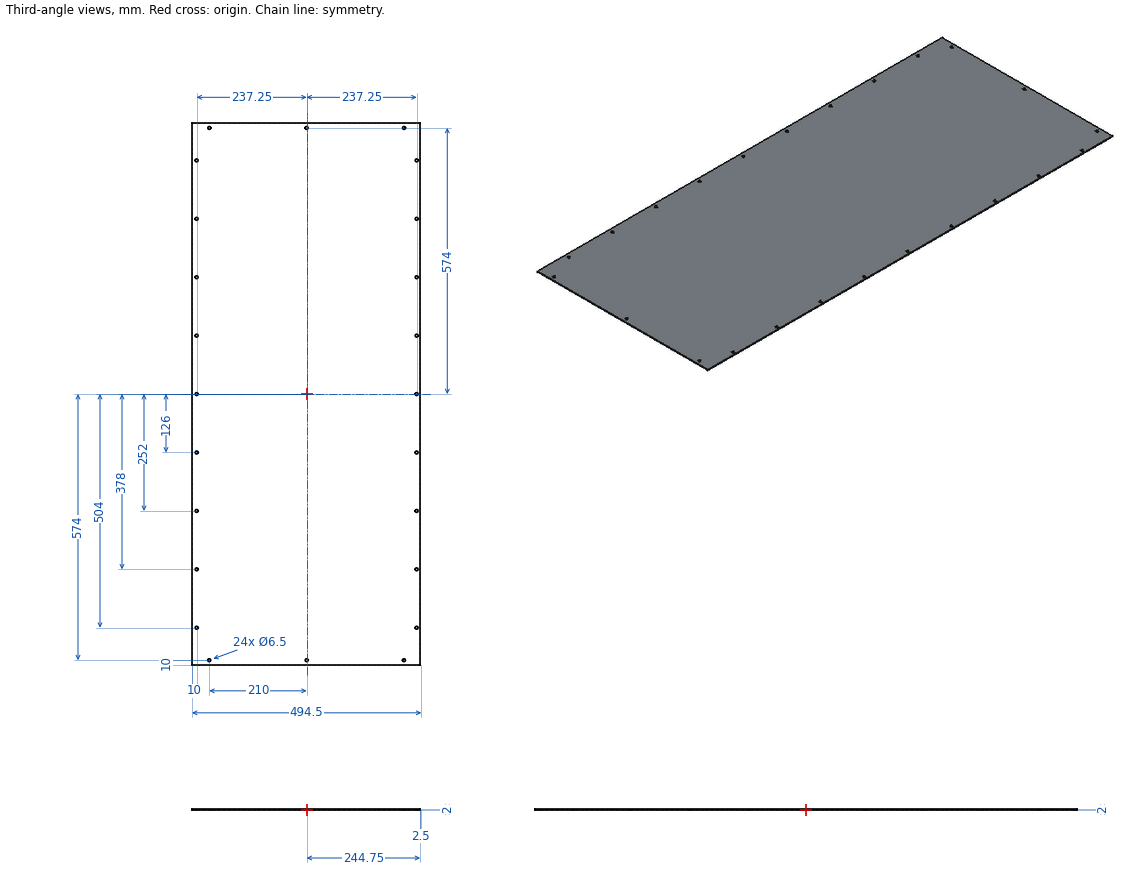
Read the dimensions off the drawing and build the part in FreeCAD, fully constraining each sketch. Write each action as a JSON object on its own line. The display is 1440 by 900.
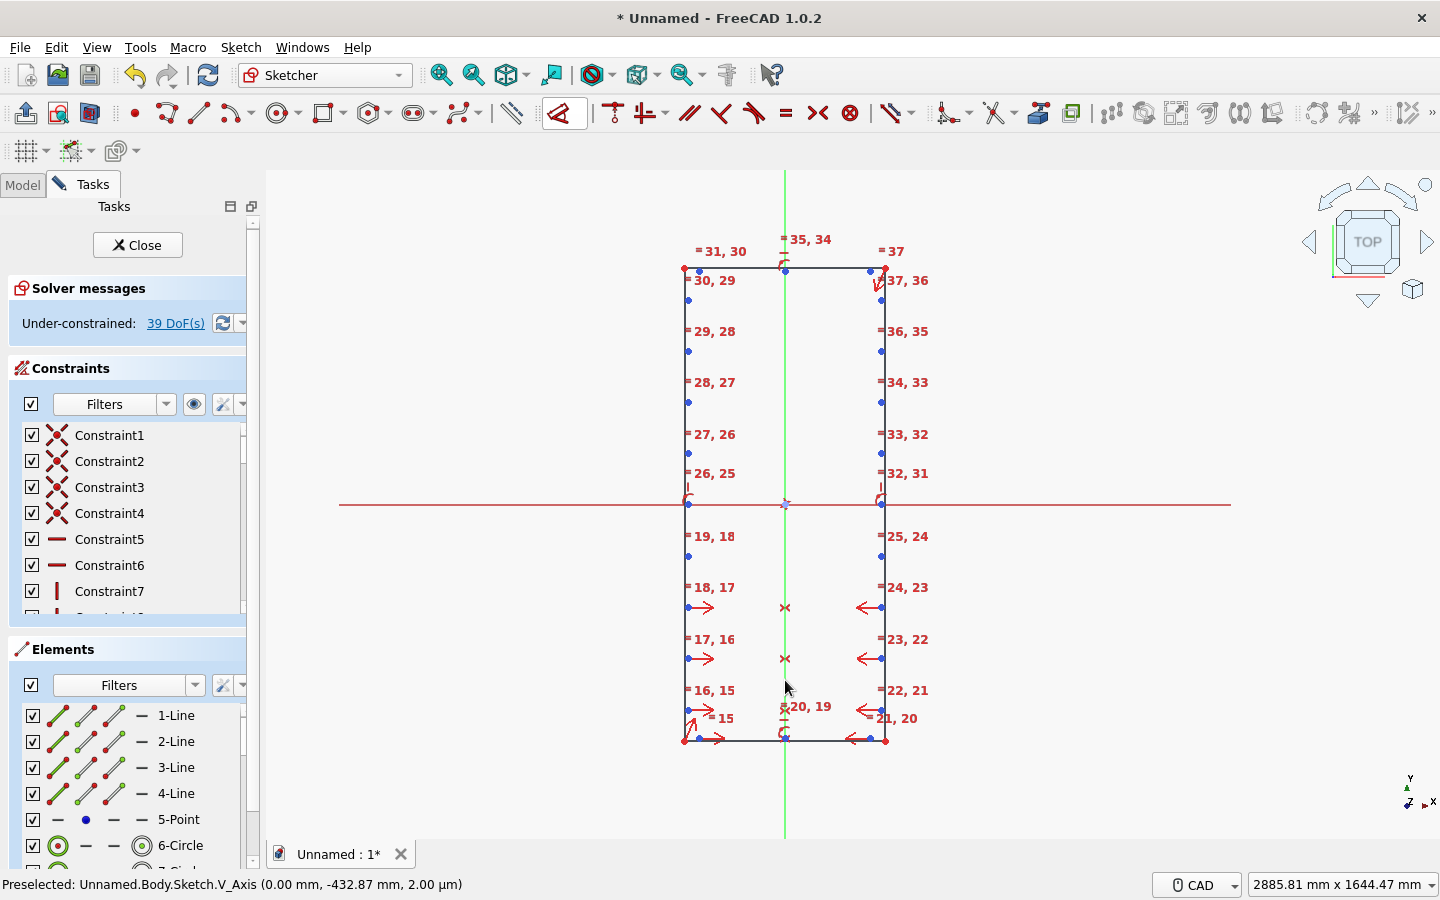
{"action": "left_click", "coordinate": [689, 556]}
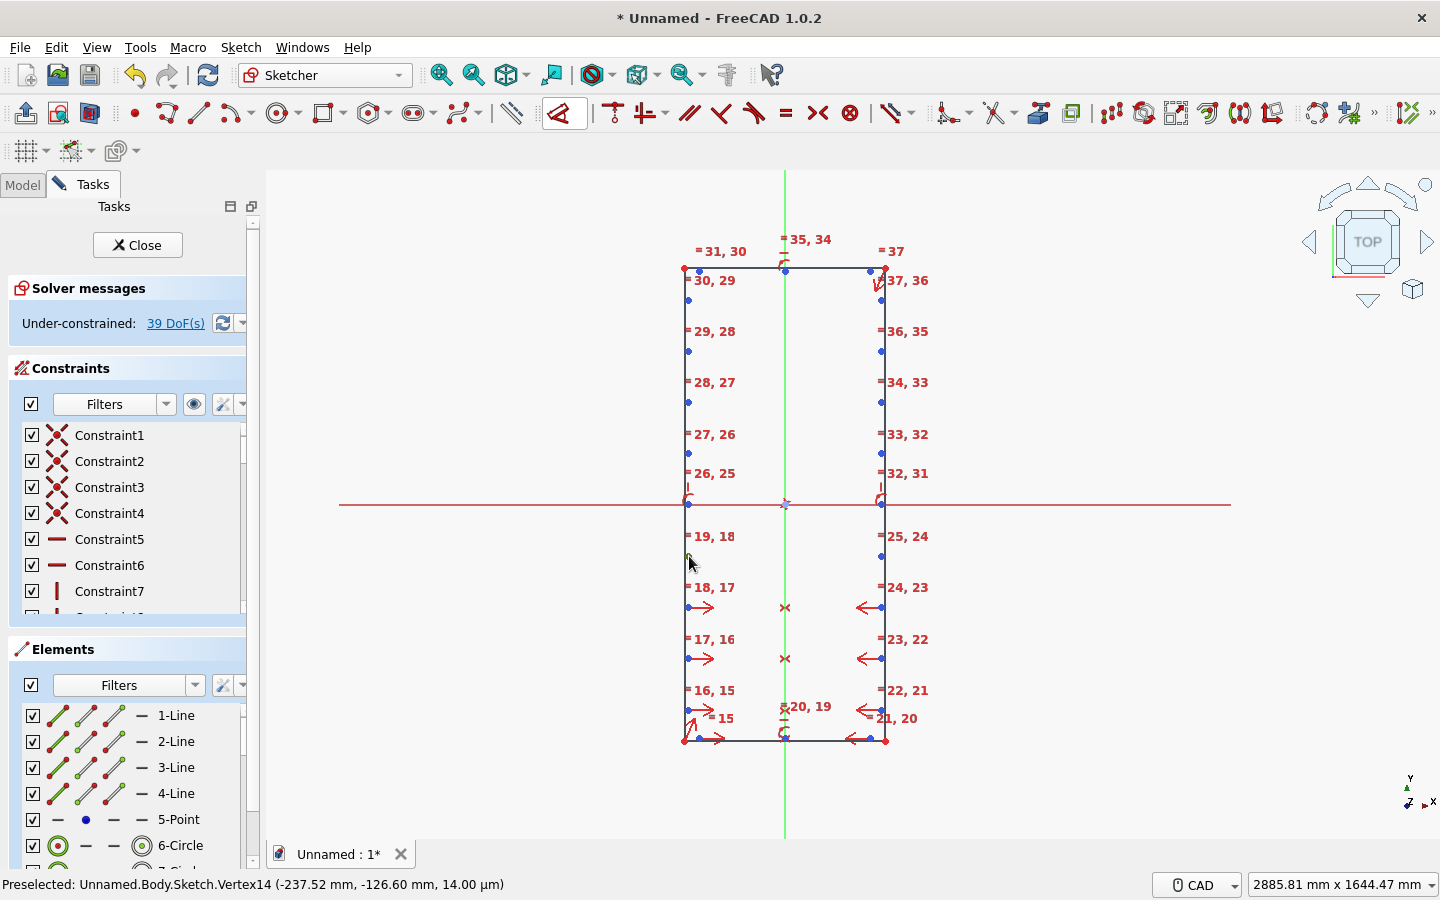
{"action": "left_click", "coordinate": [882, 556]}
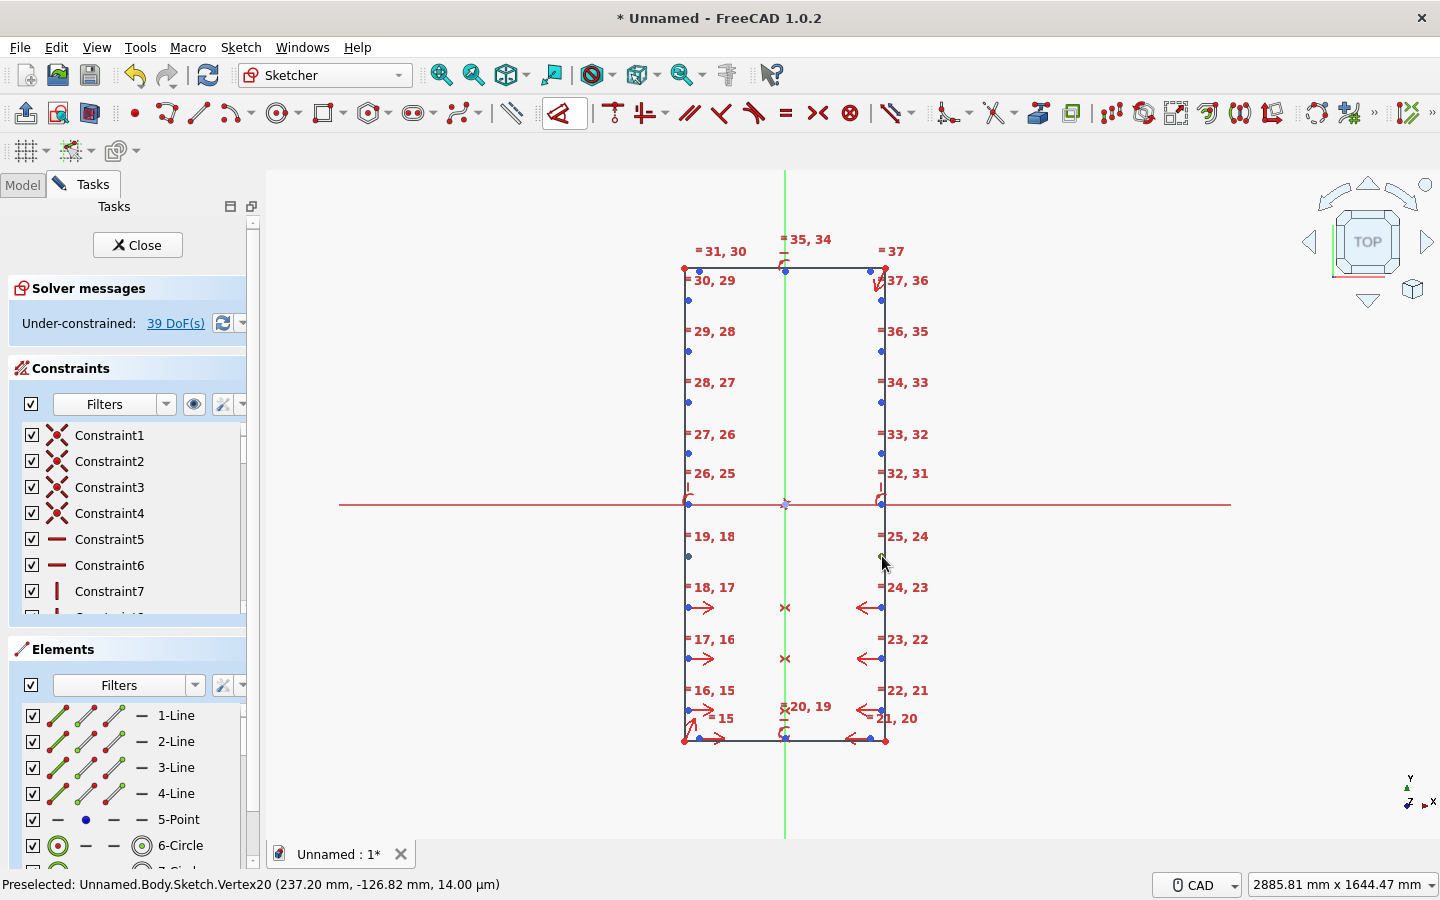
{"action": "left_click", "coordinate": [785, 680]}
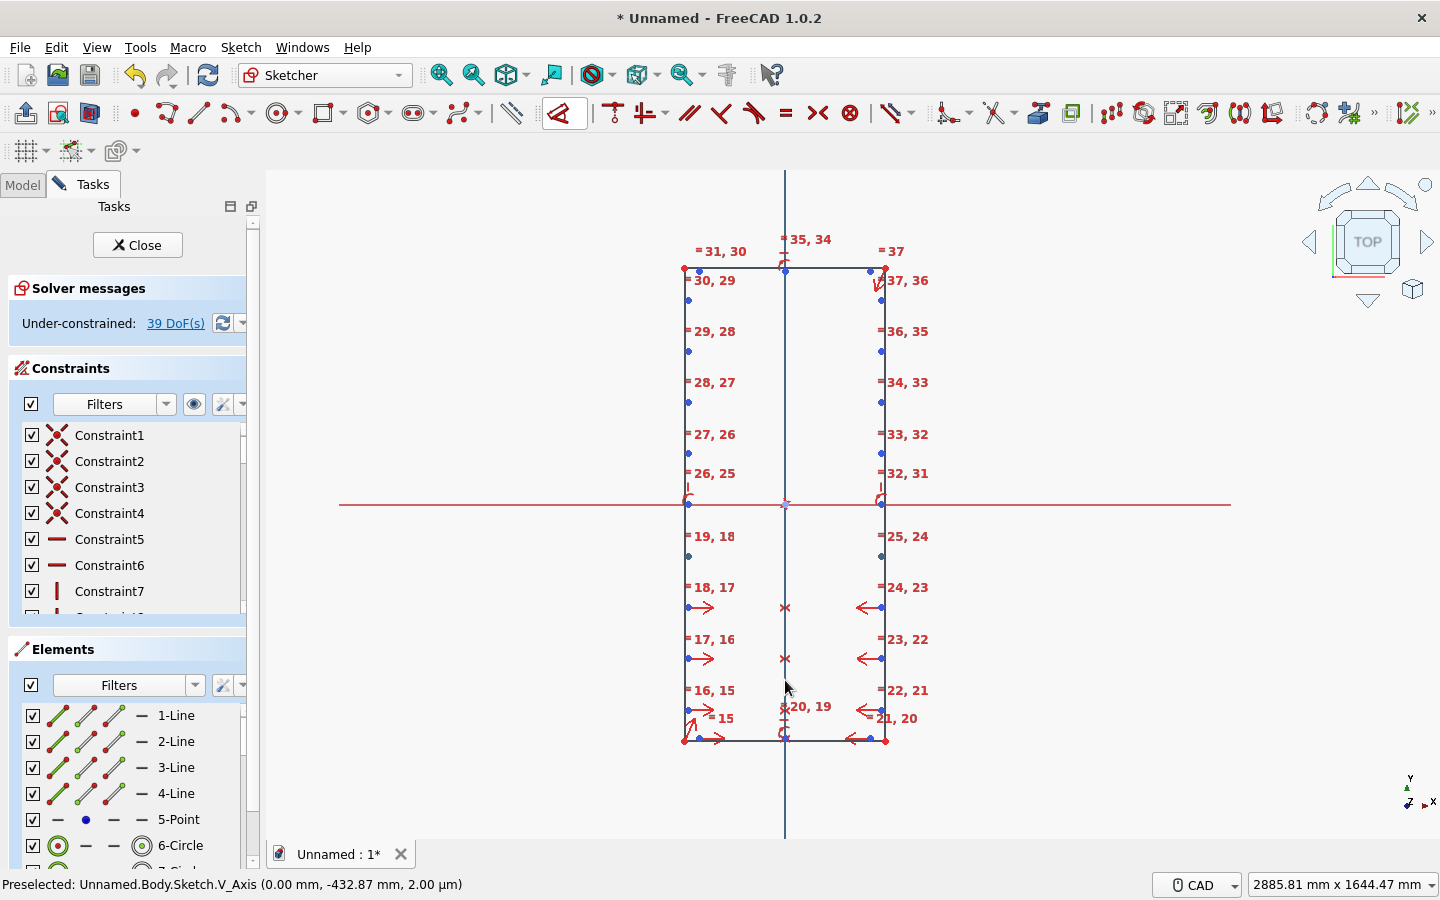
{"action": "left_click", "coordinate": [818, 114]}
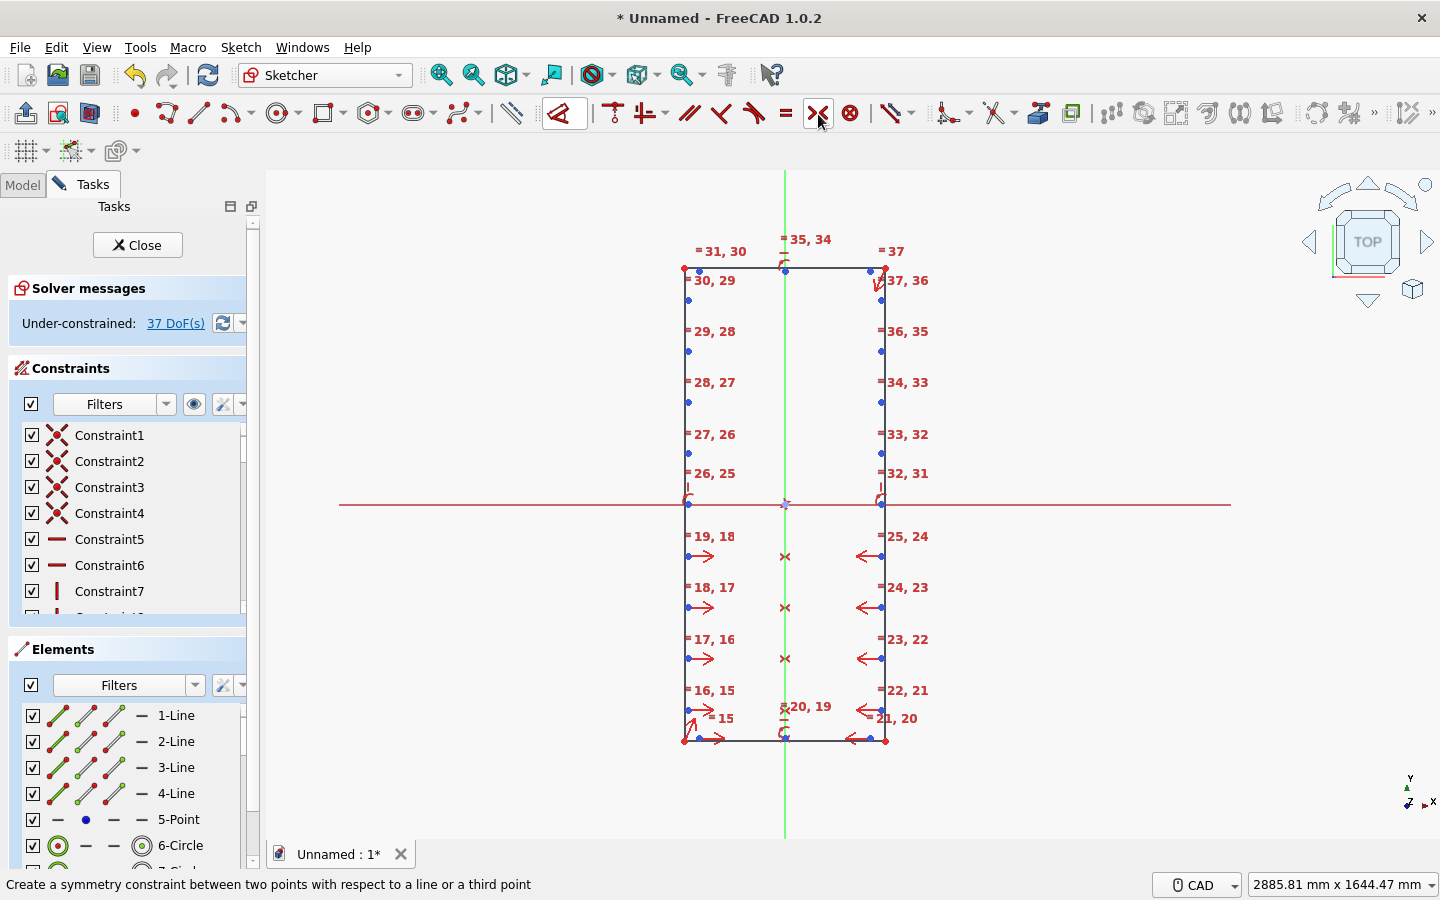
{"action": "left_click", "coordinate": [689, 556]}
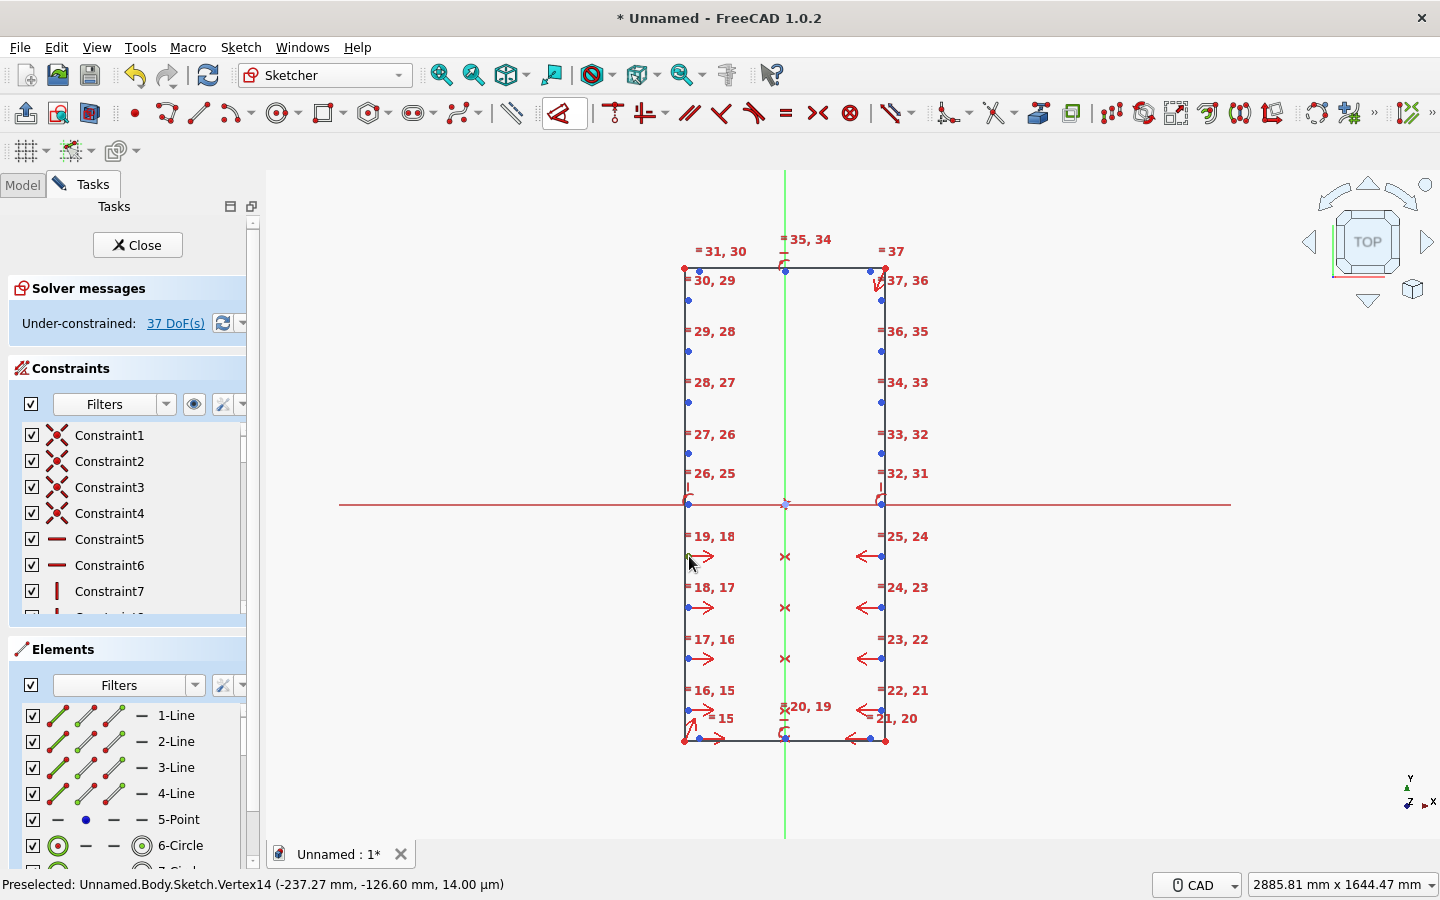
{"action": "left_click", "coordinate": [689, 454]}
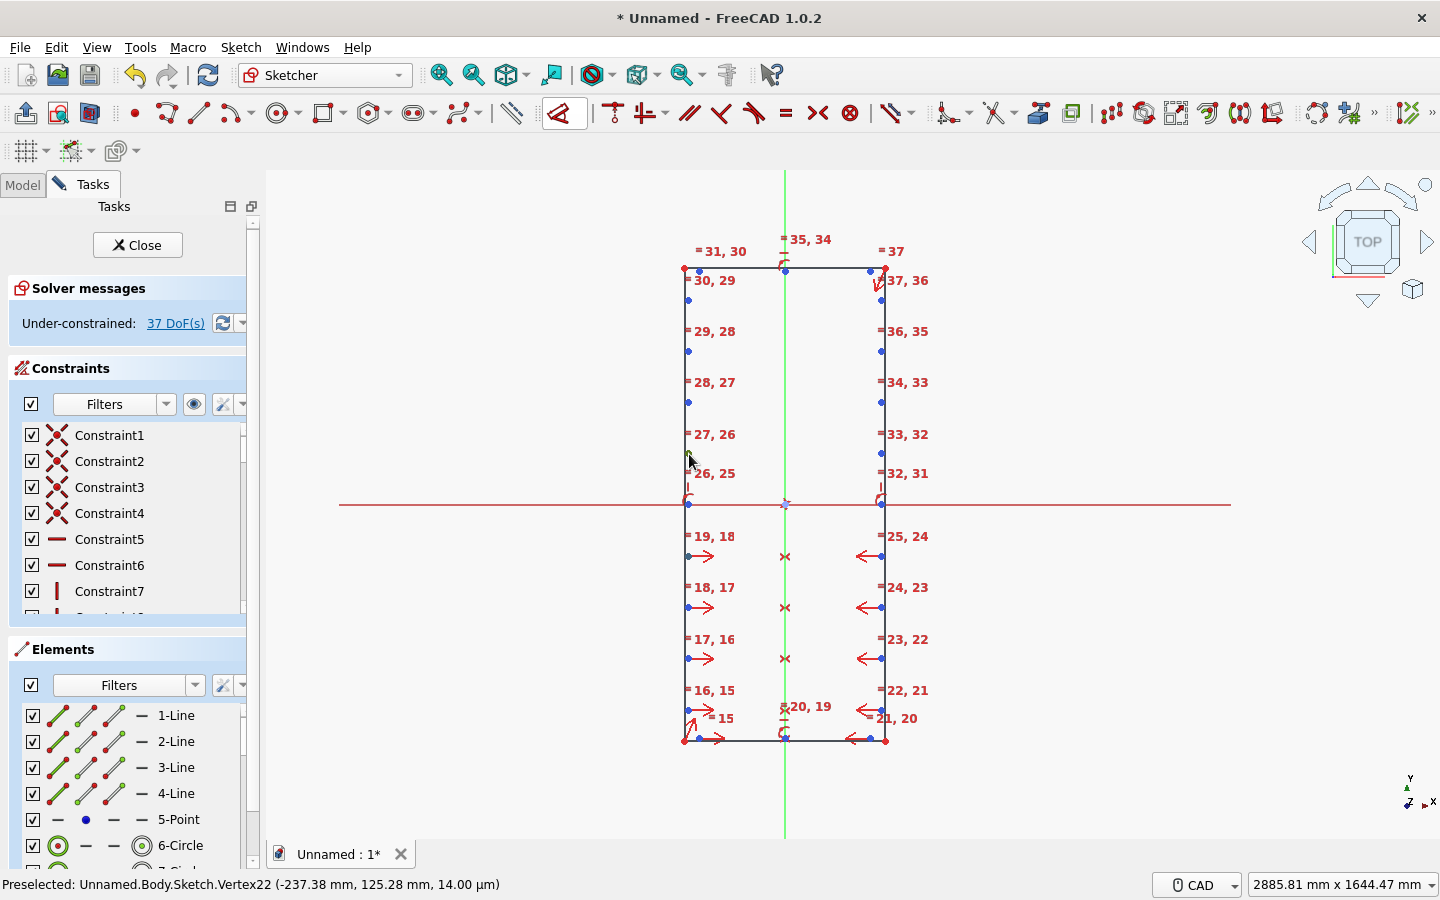
{"action": "left_click", "coordinate": [364, 505]}